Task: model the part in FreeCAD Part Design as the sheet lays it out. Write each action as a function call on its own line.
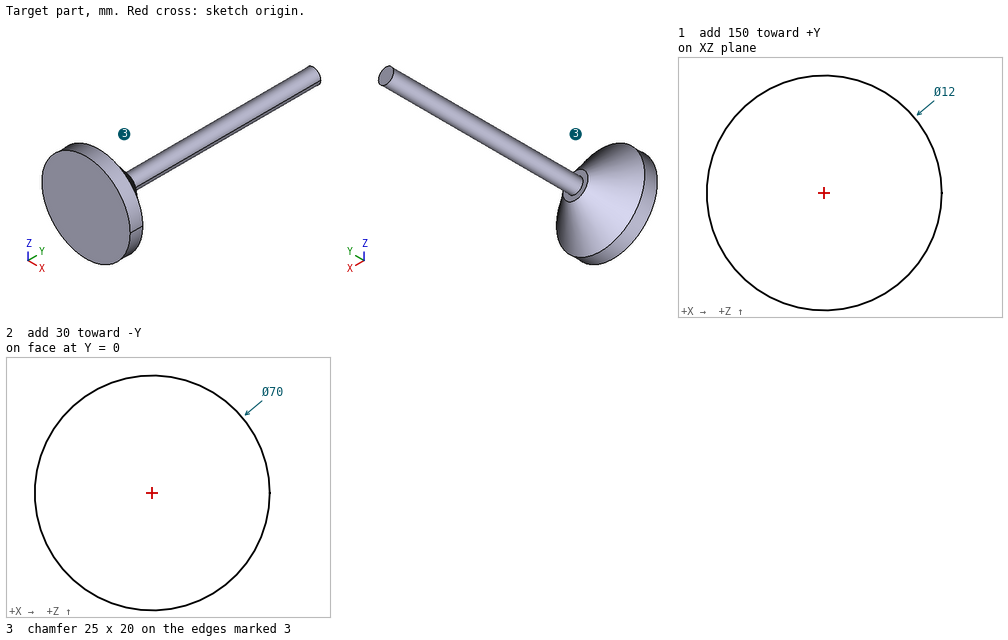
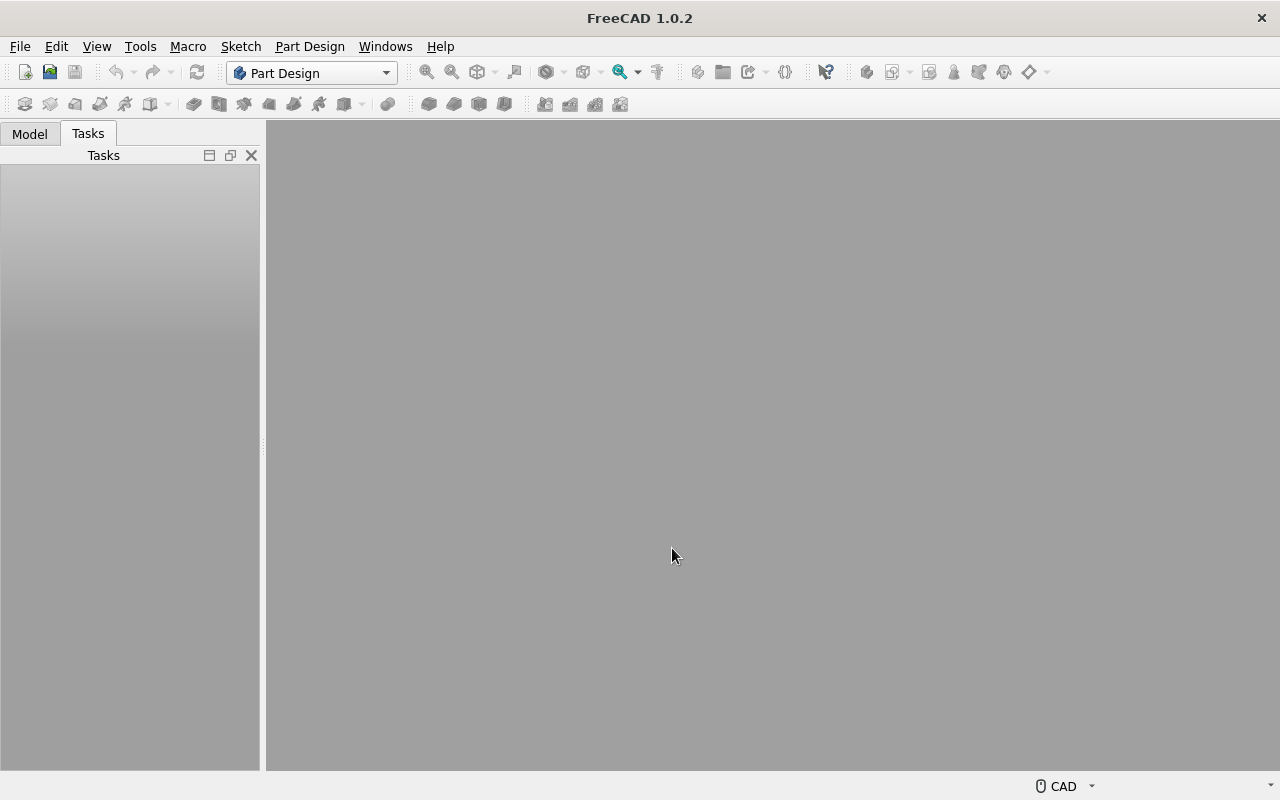
click(25, 72)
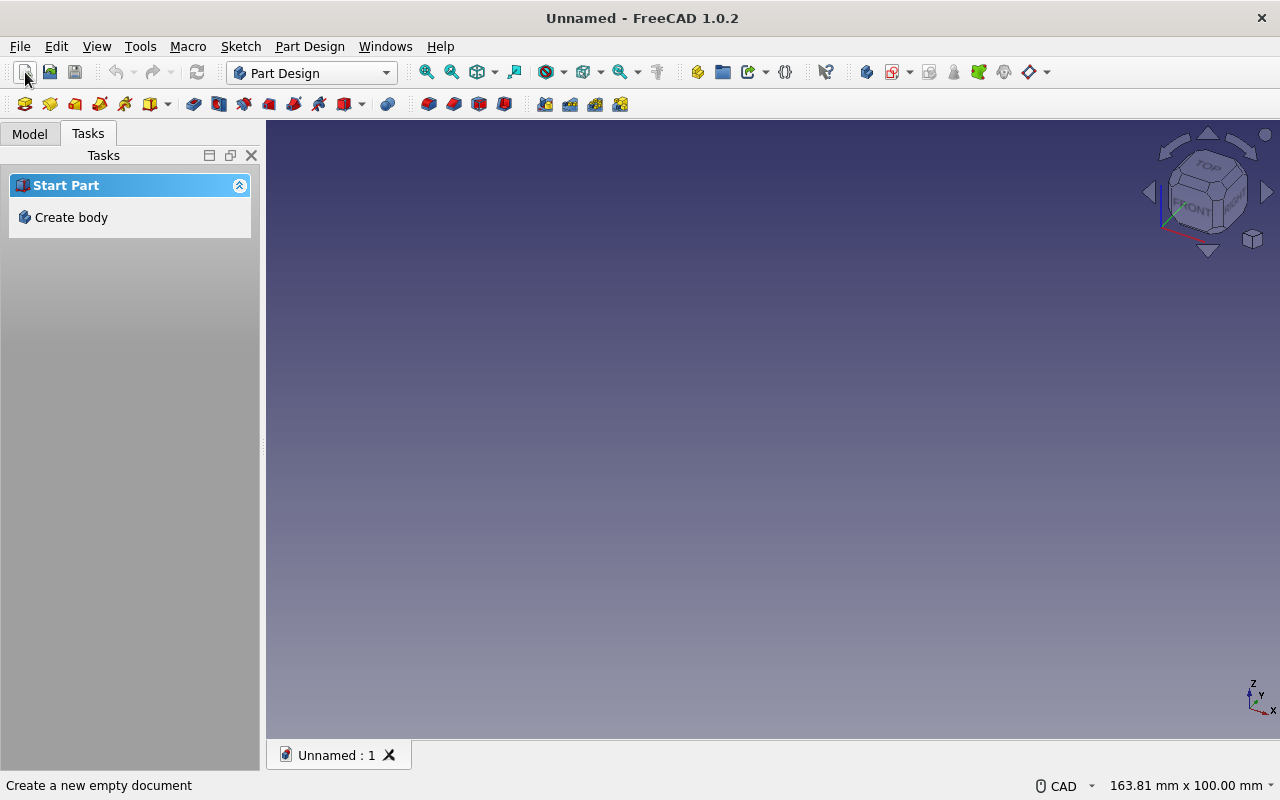
click(892, 72)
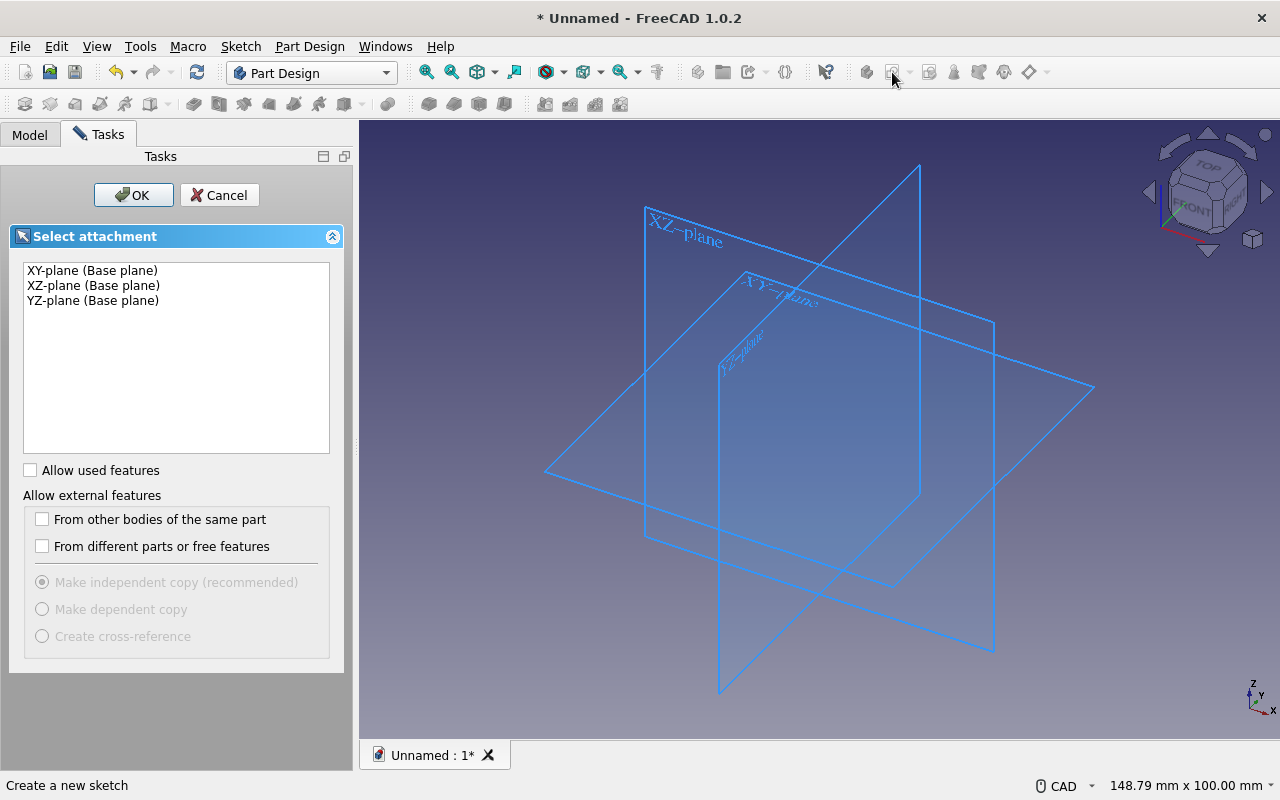
click(84, 286)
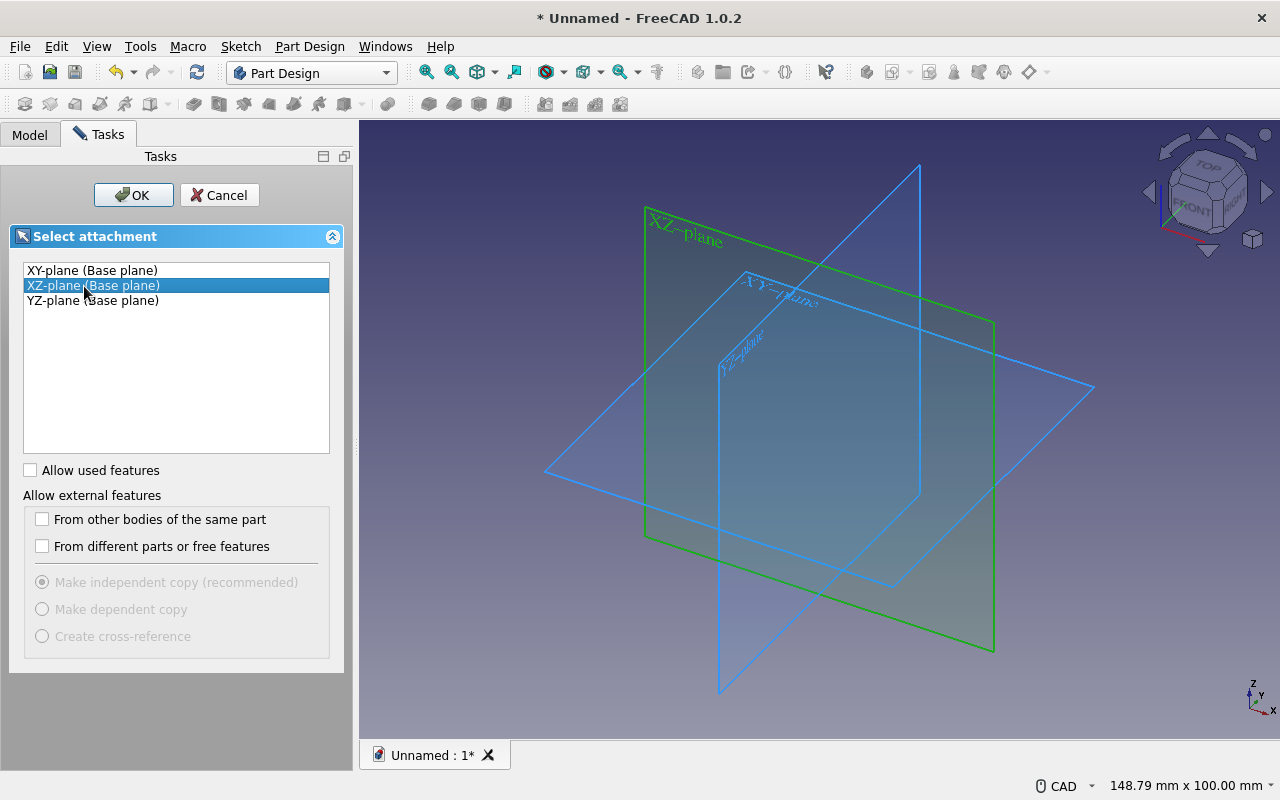
click(134, 195)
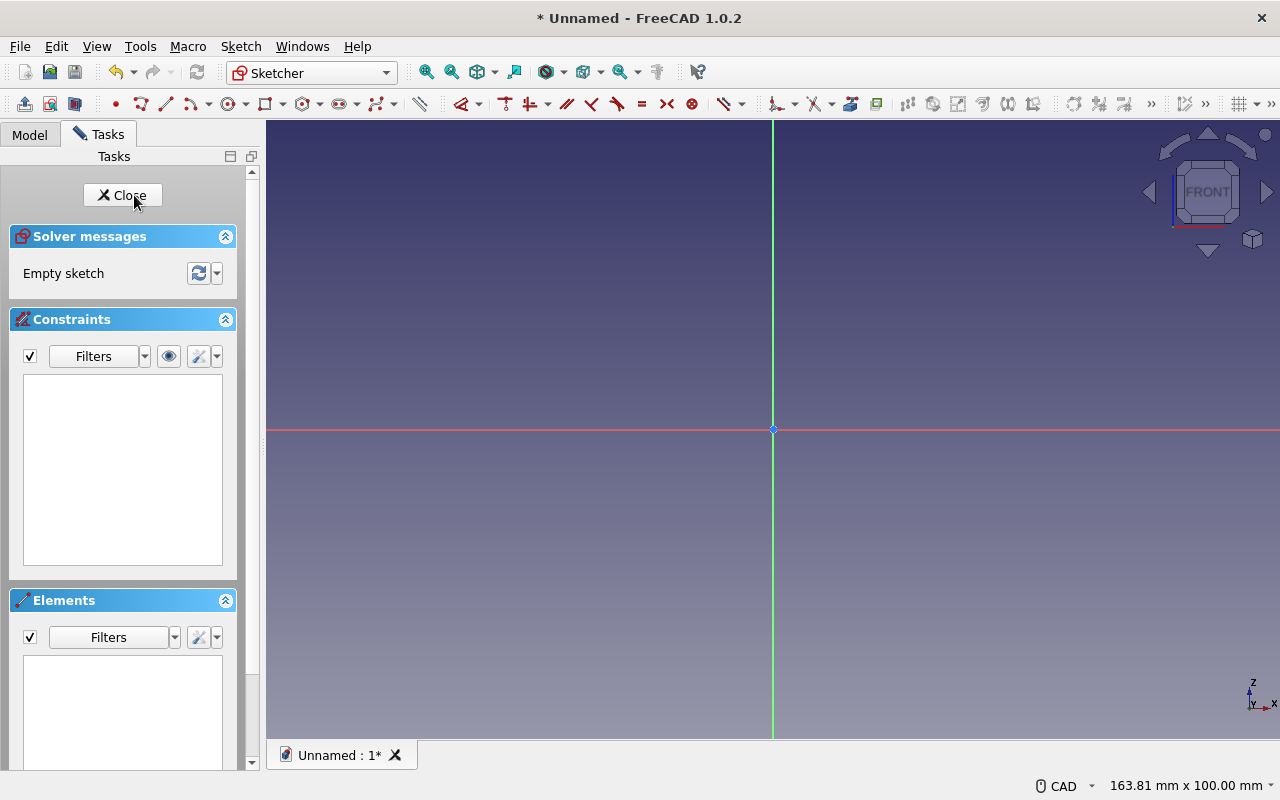
scroll(790, 430, up, 8)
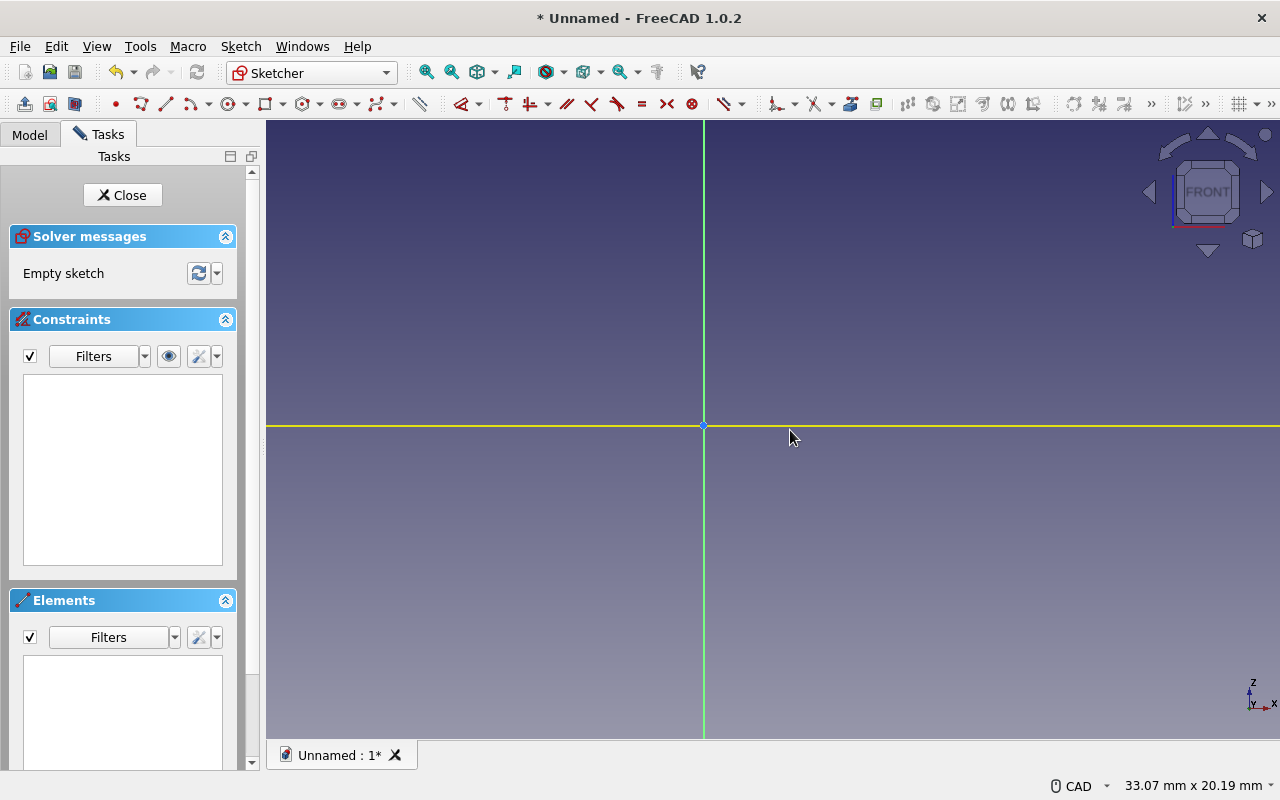
click(228, 104)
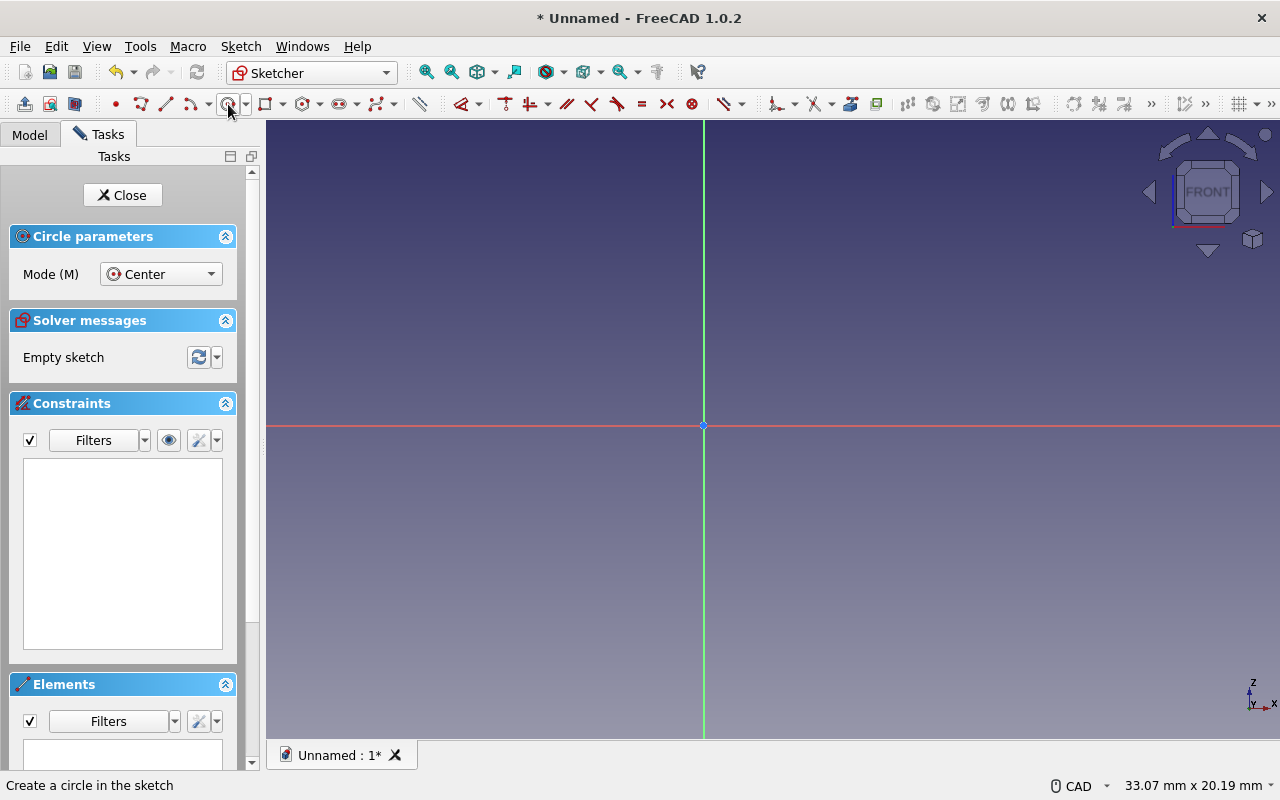
click(704, 426)
click(834, 295)
key(Escape)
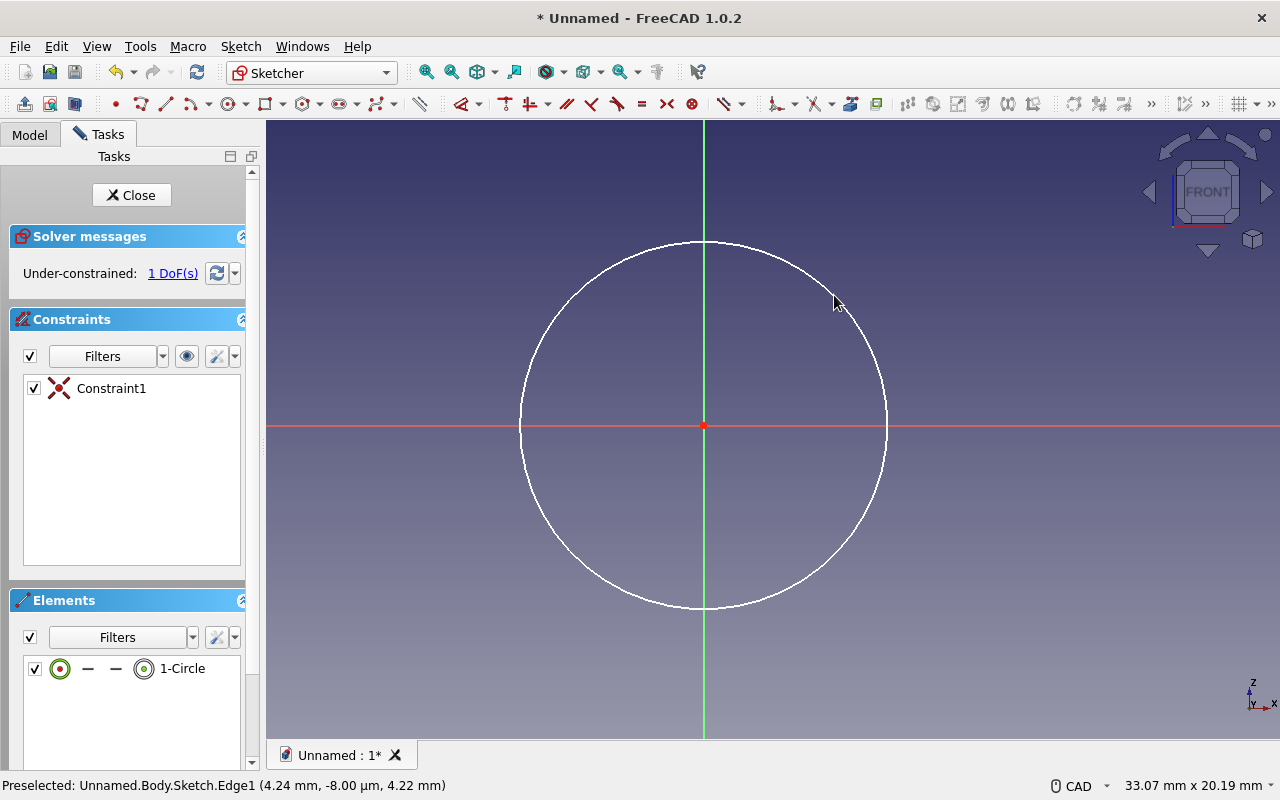
click(833, 295)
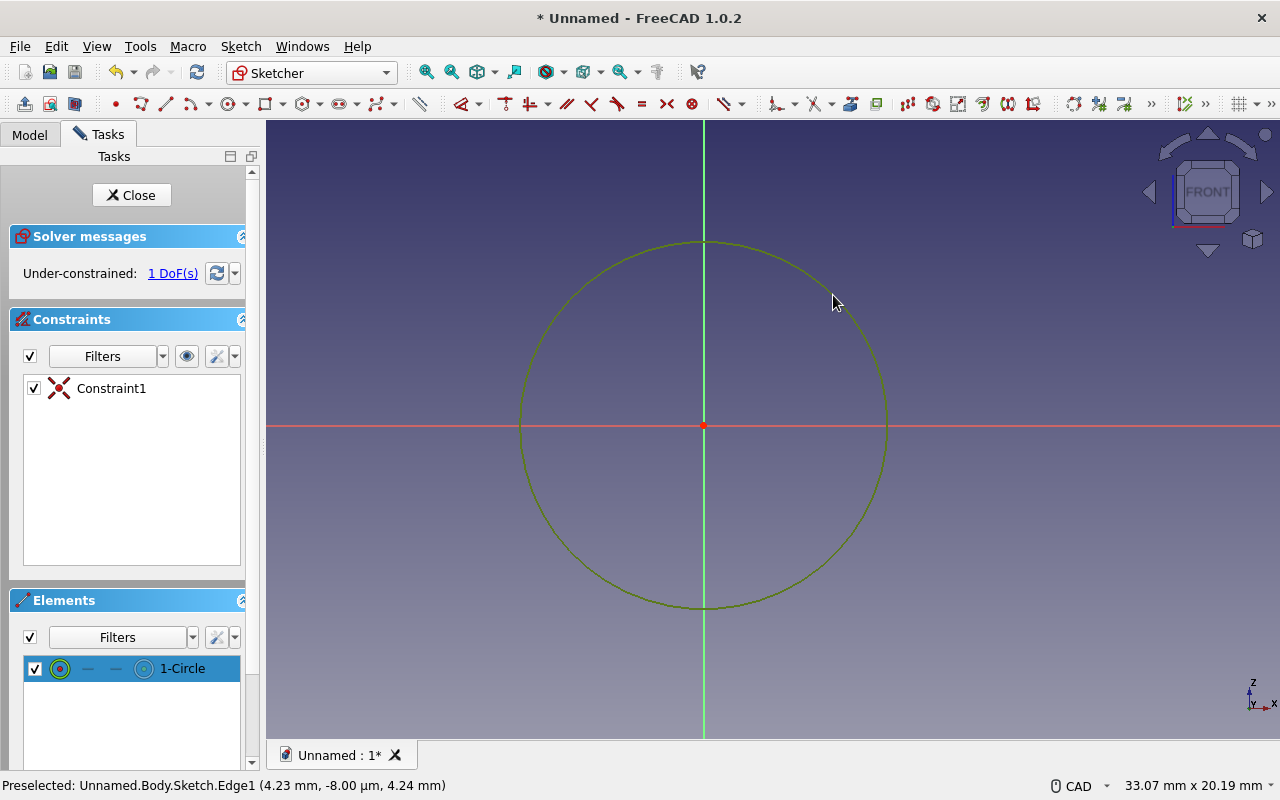
click(478, 104)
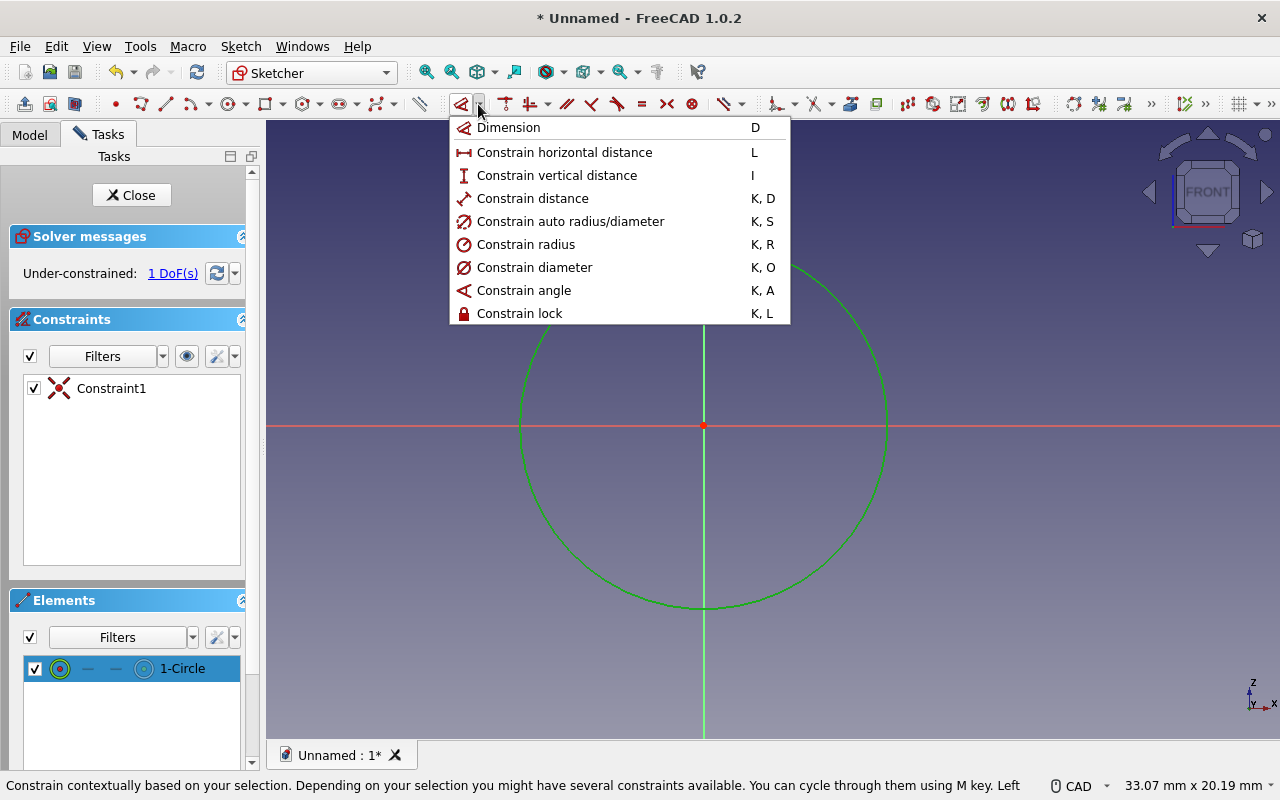
click(620, 268)